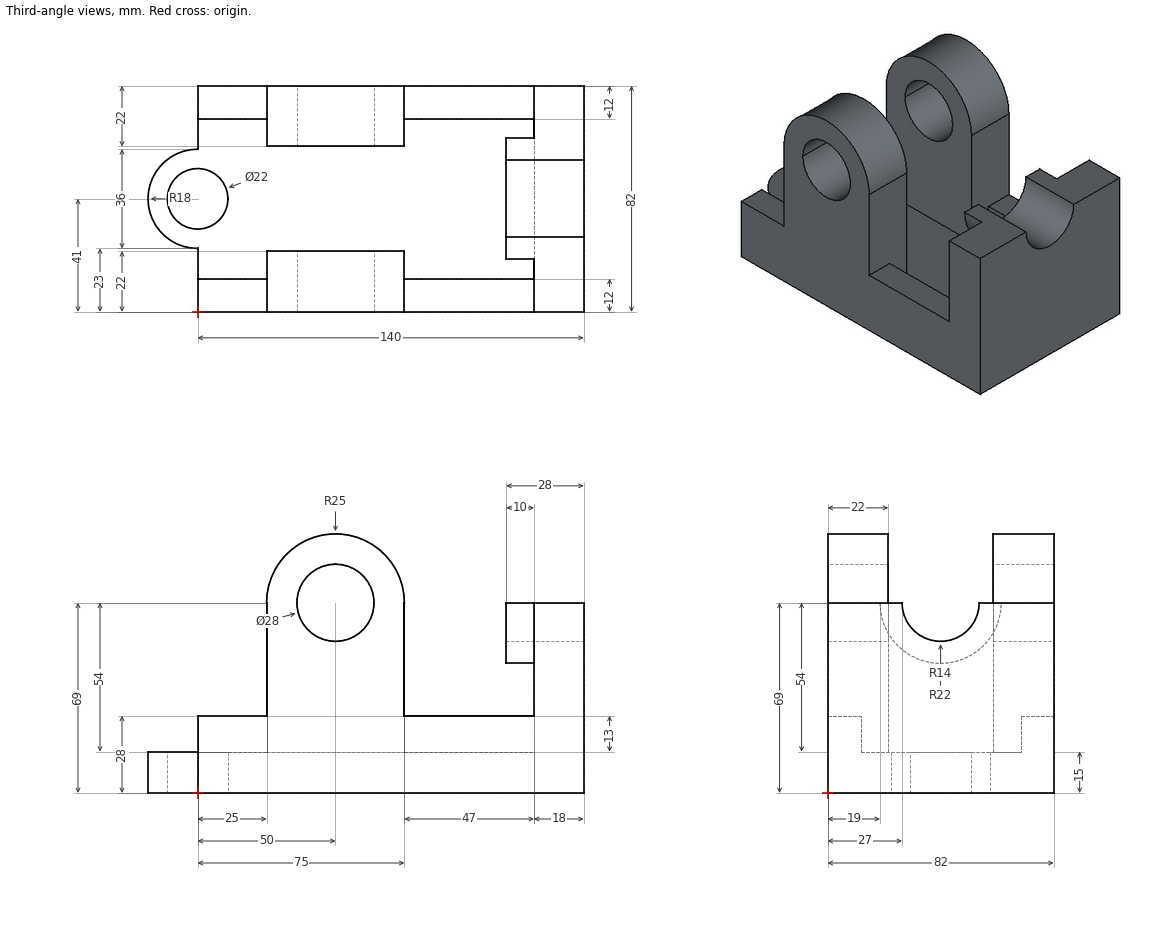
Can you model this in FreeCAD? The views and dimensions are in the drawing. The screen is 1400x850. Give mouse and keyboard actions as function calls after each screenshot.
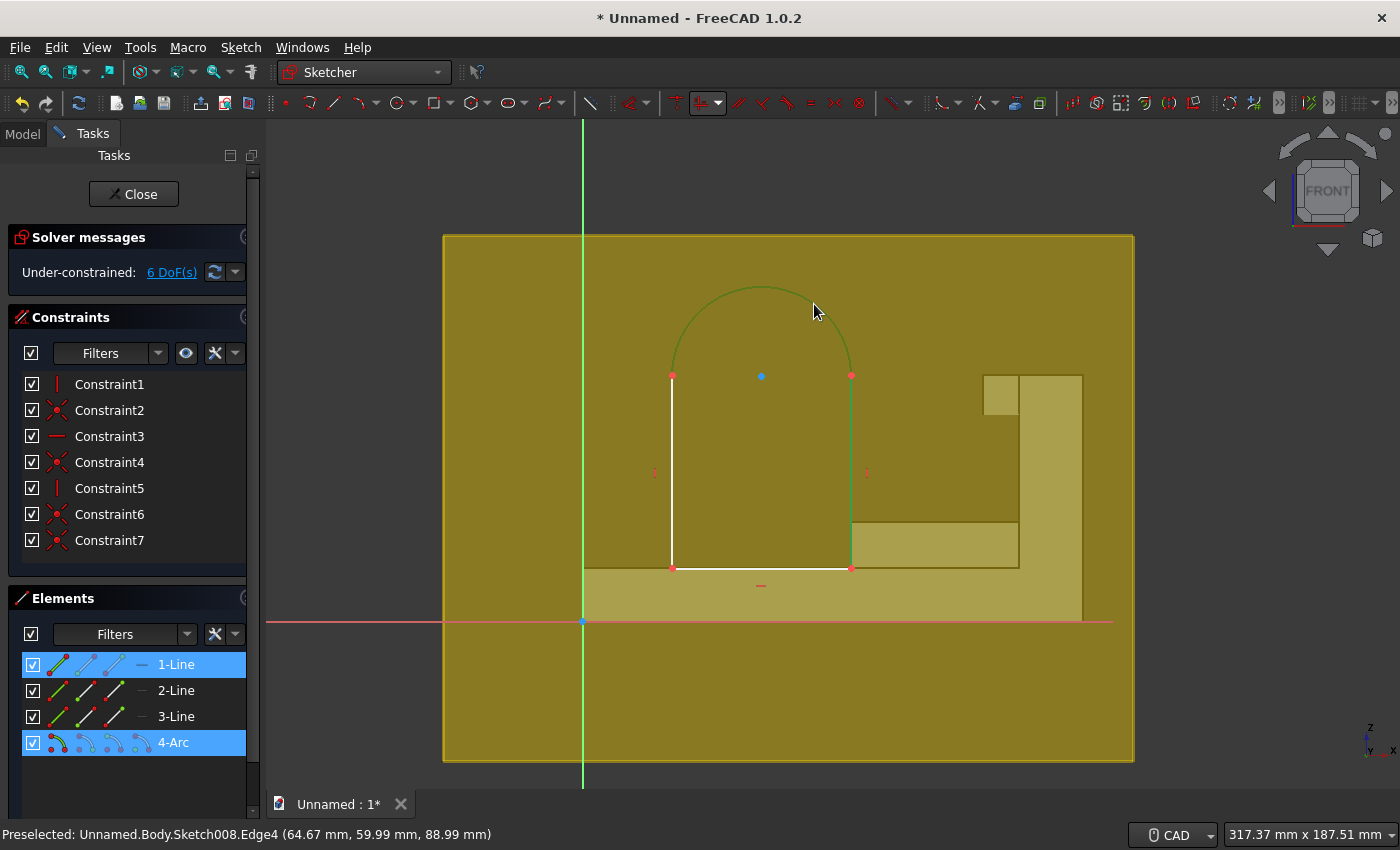
click(788, 104)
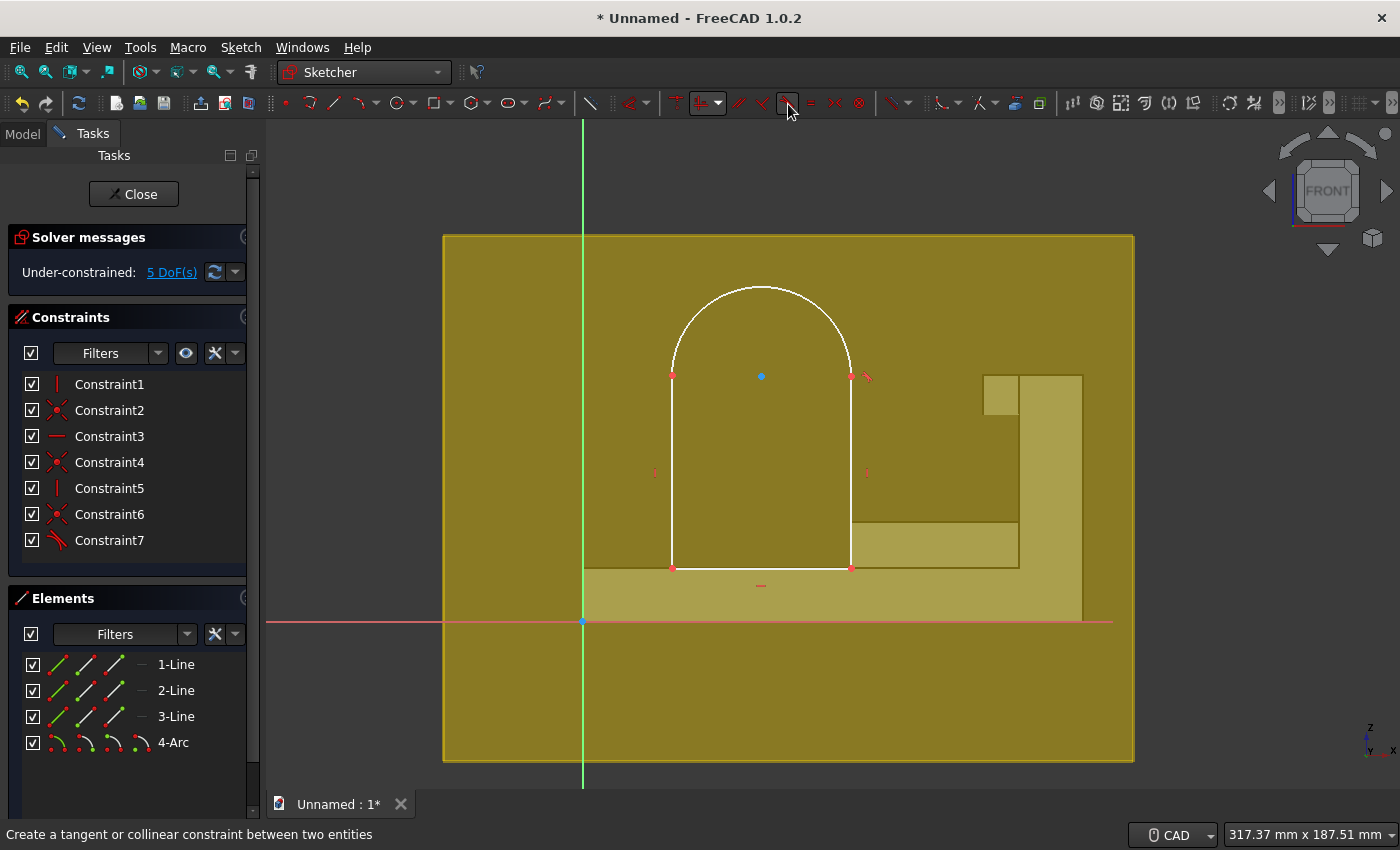
click(672, 511)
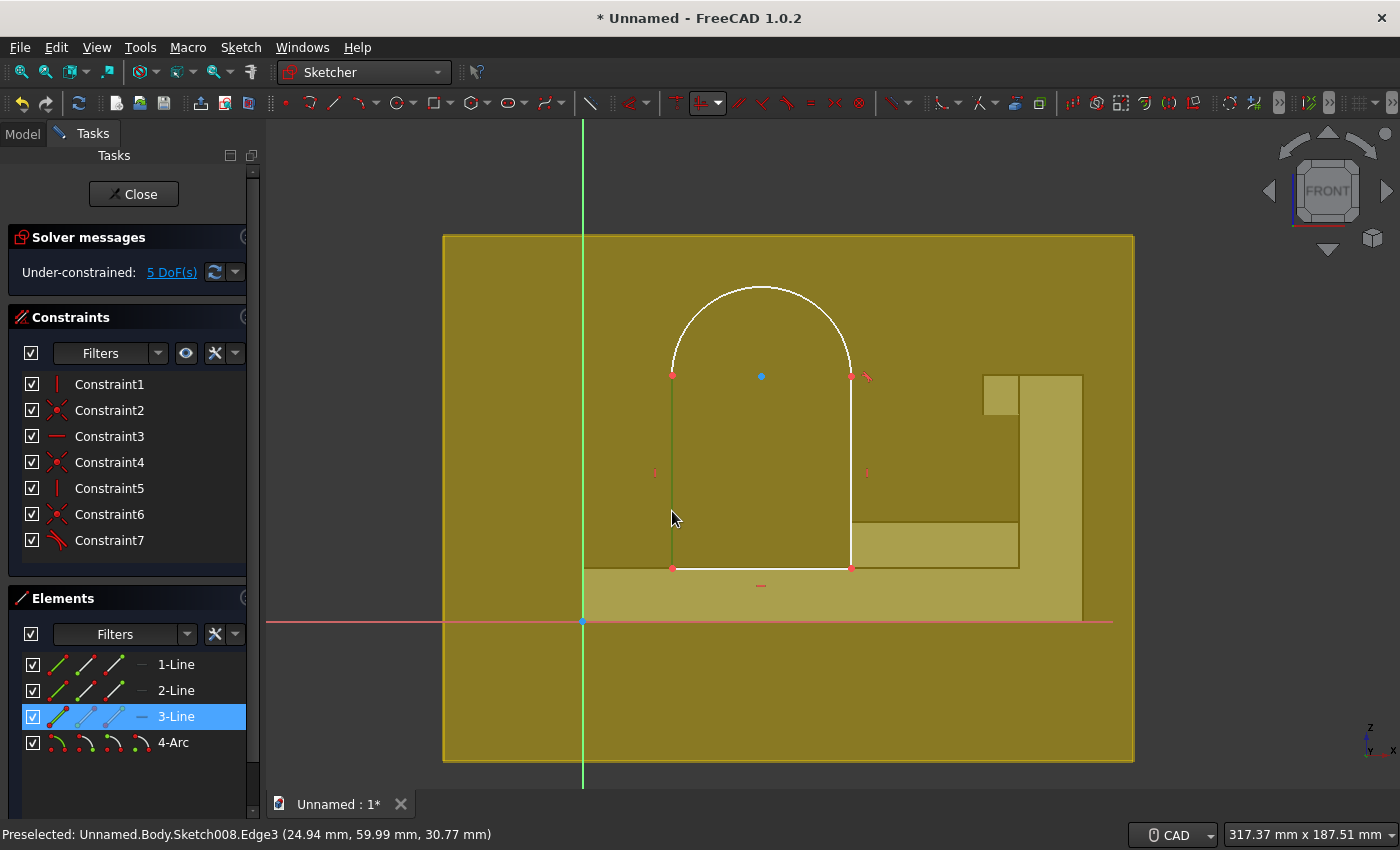
click(814, 304)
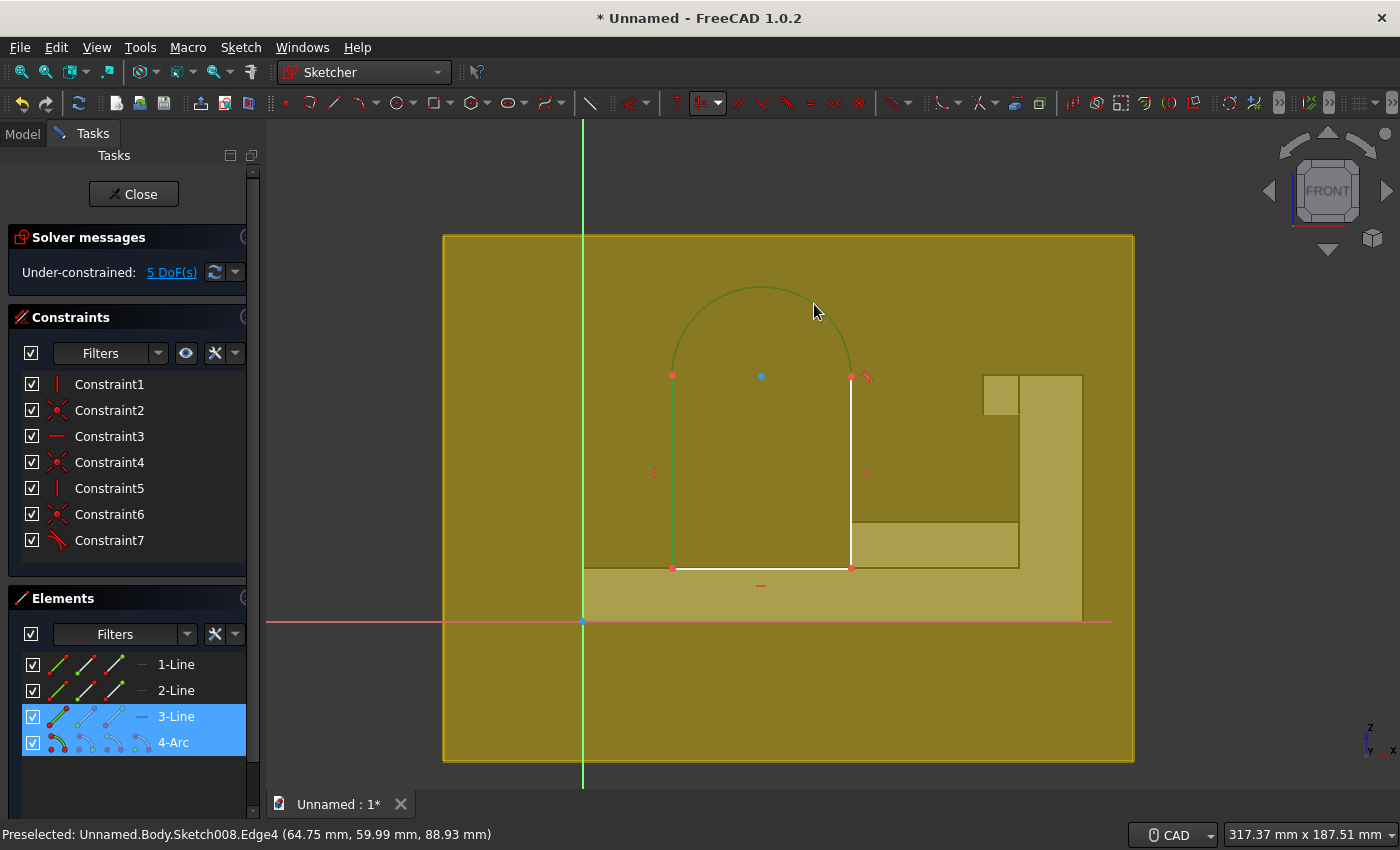
click(788, 104)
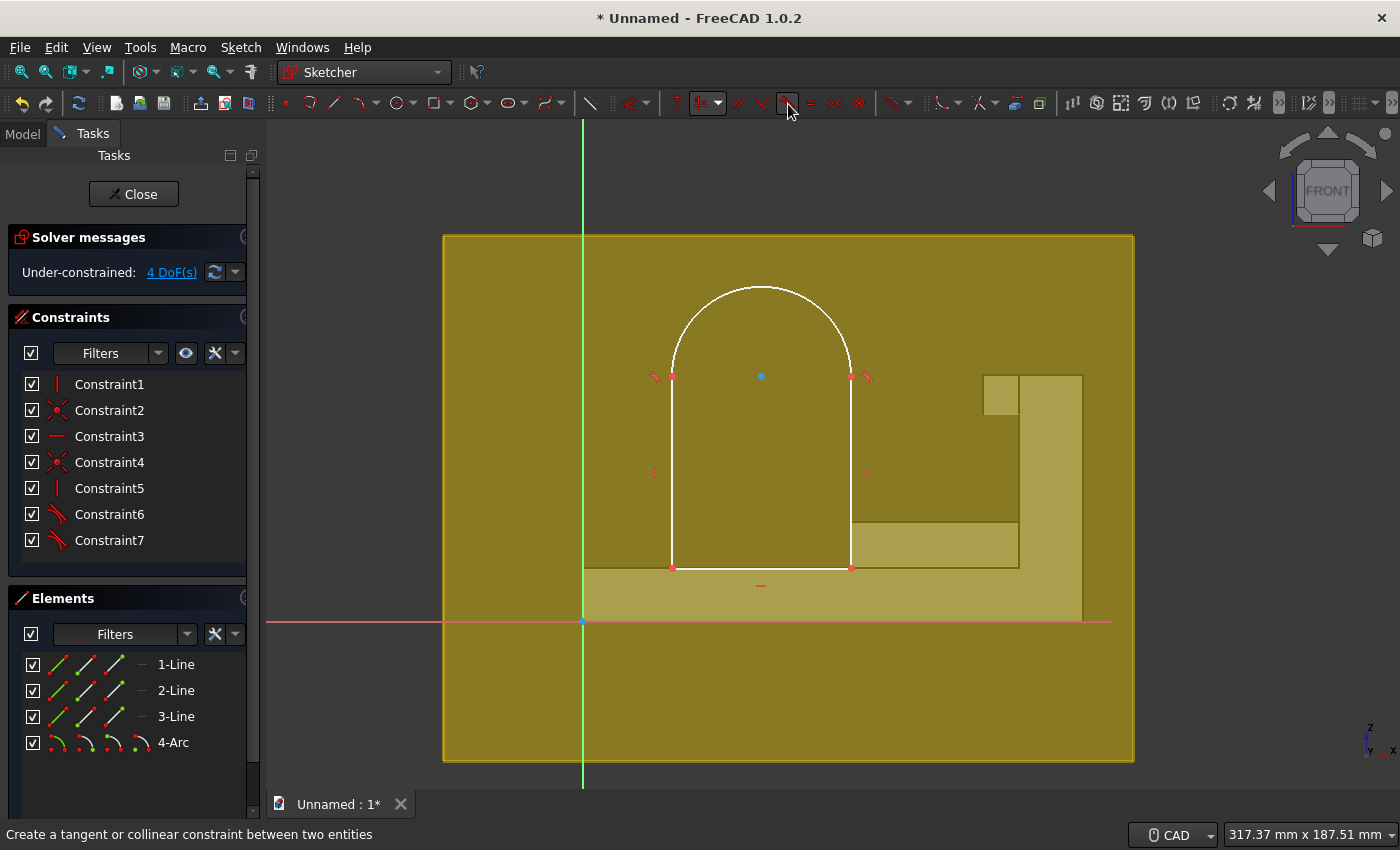
click(630, 104)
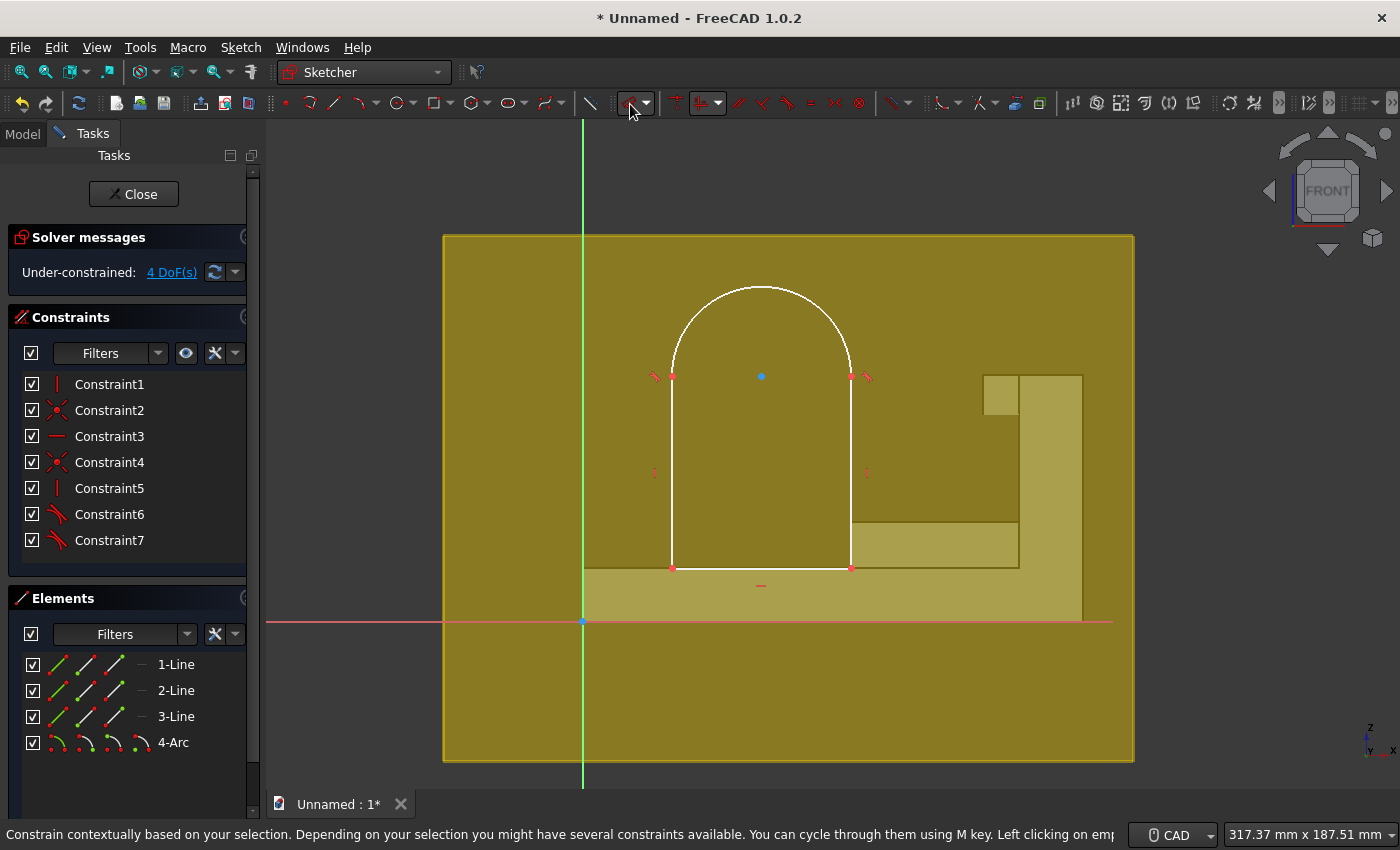
click(814, 304)
click(833, 278)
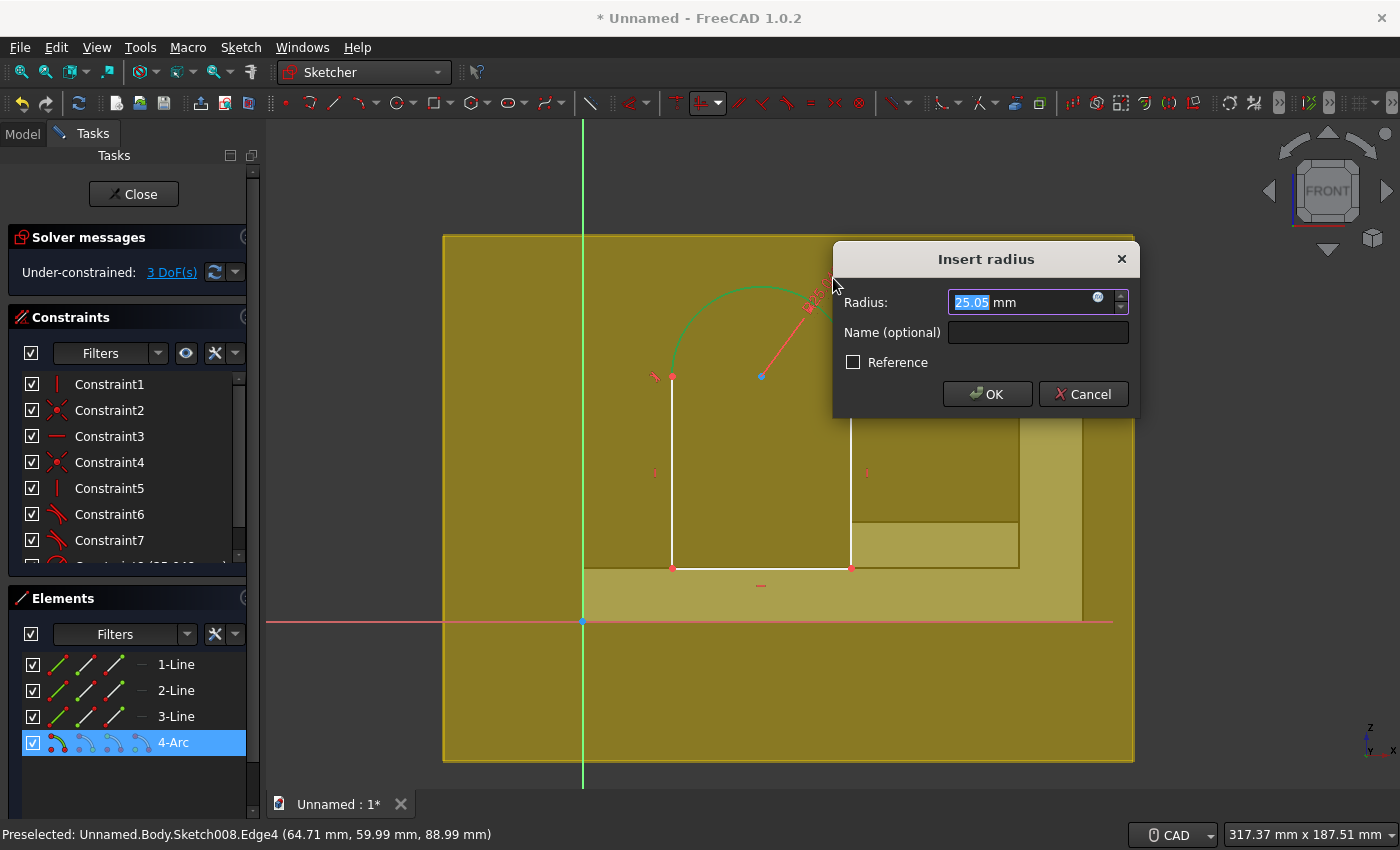
text(25)
key(Return)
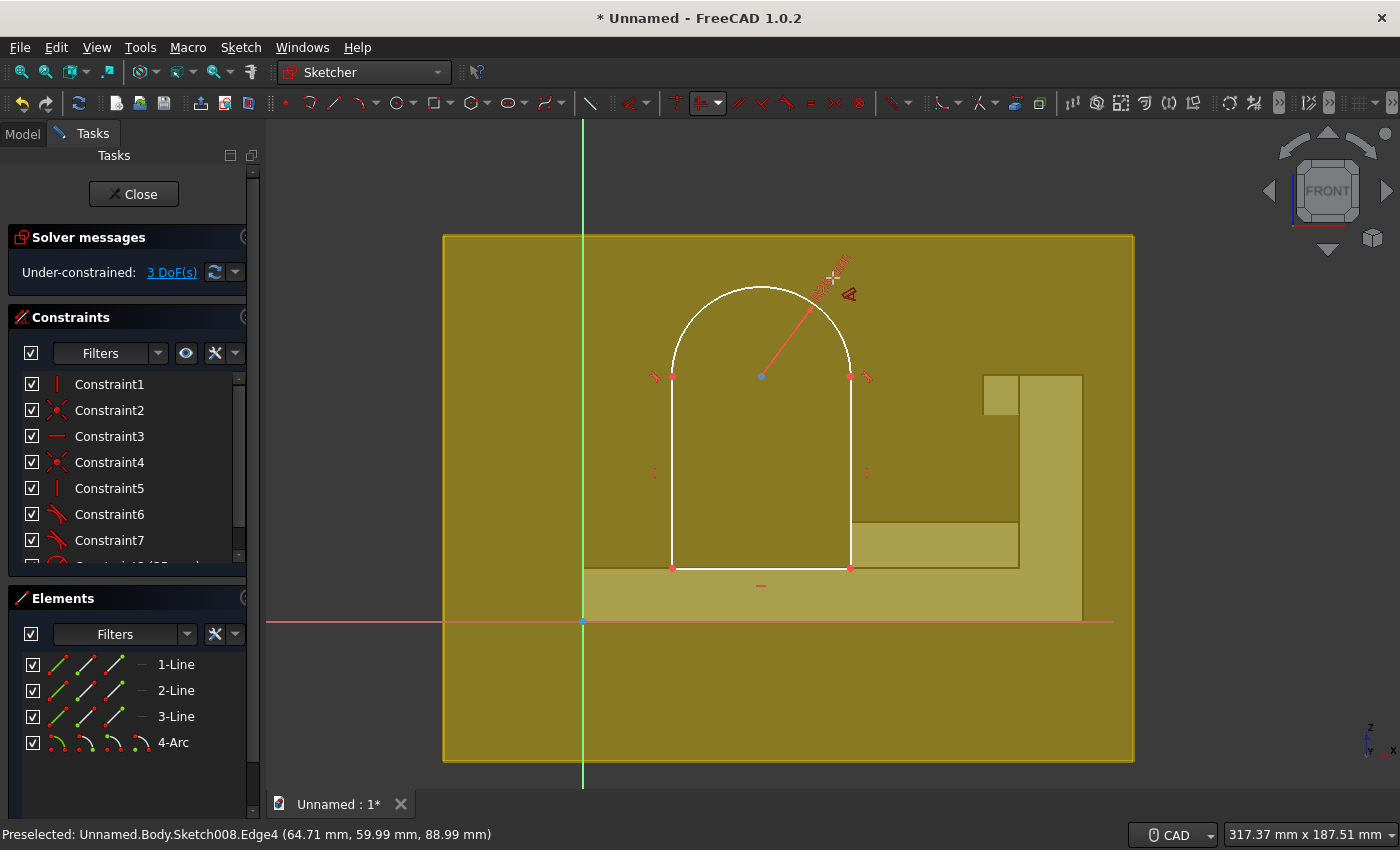
click(851, 434)
click(885, 473)